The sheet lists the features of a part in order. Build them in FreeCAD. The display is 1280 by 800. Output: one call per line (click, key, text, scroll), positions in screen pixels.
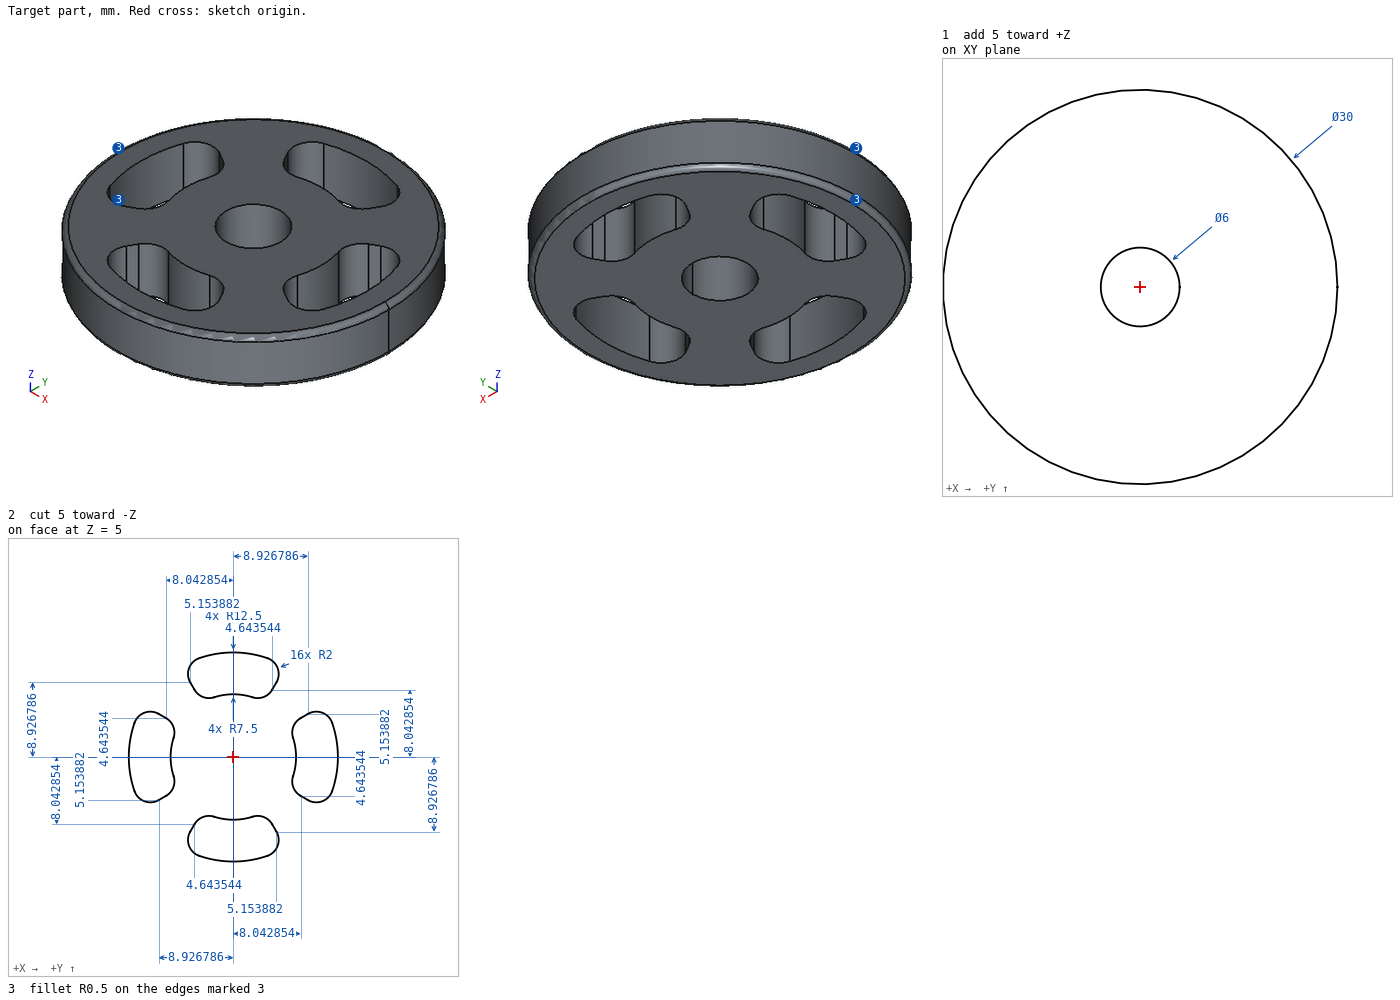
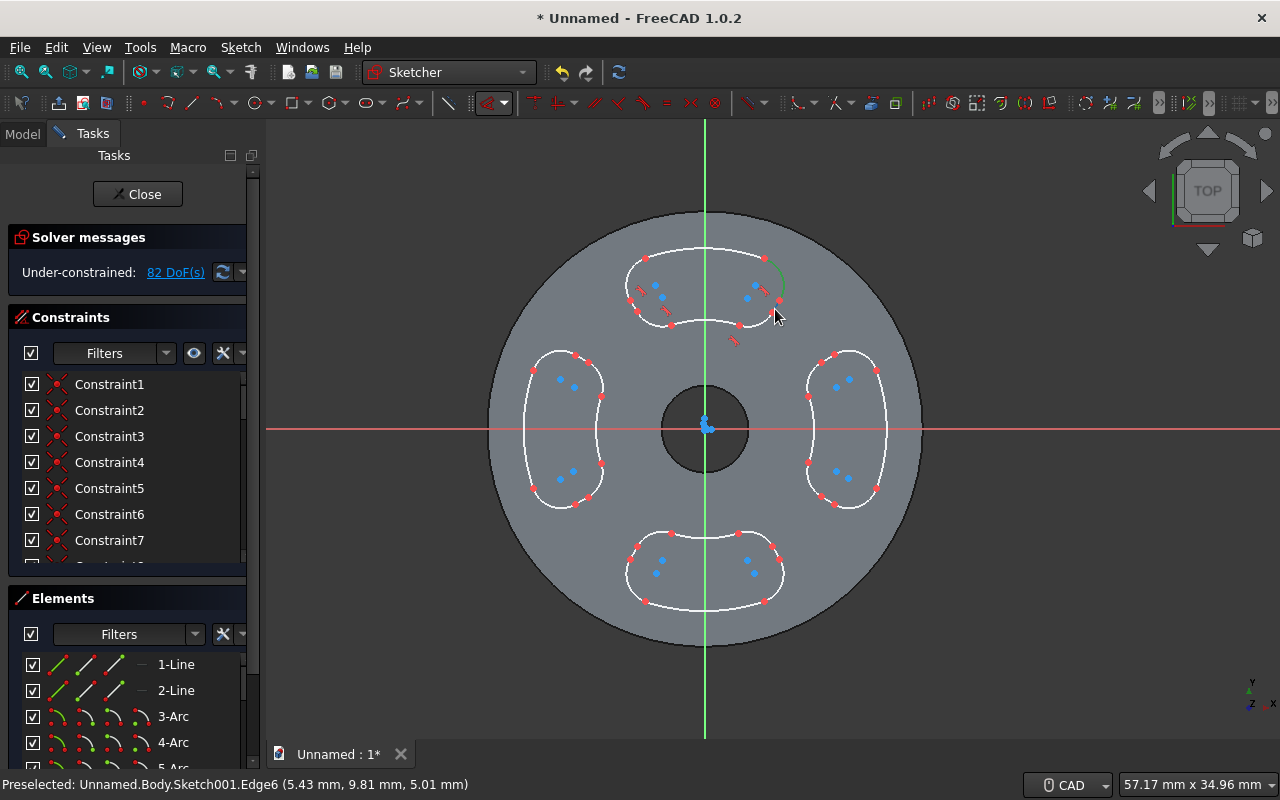
click(729, 250)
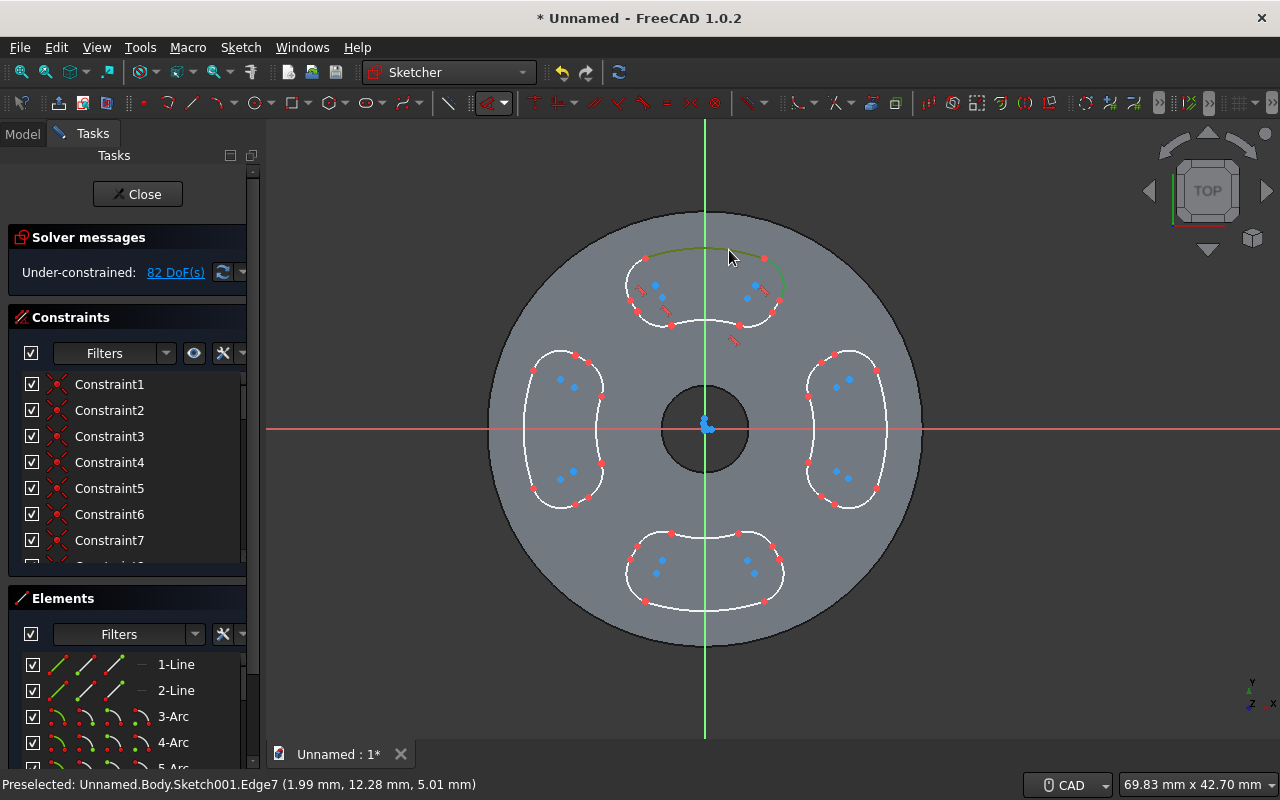
click(644, 104)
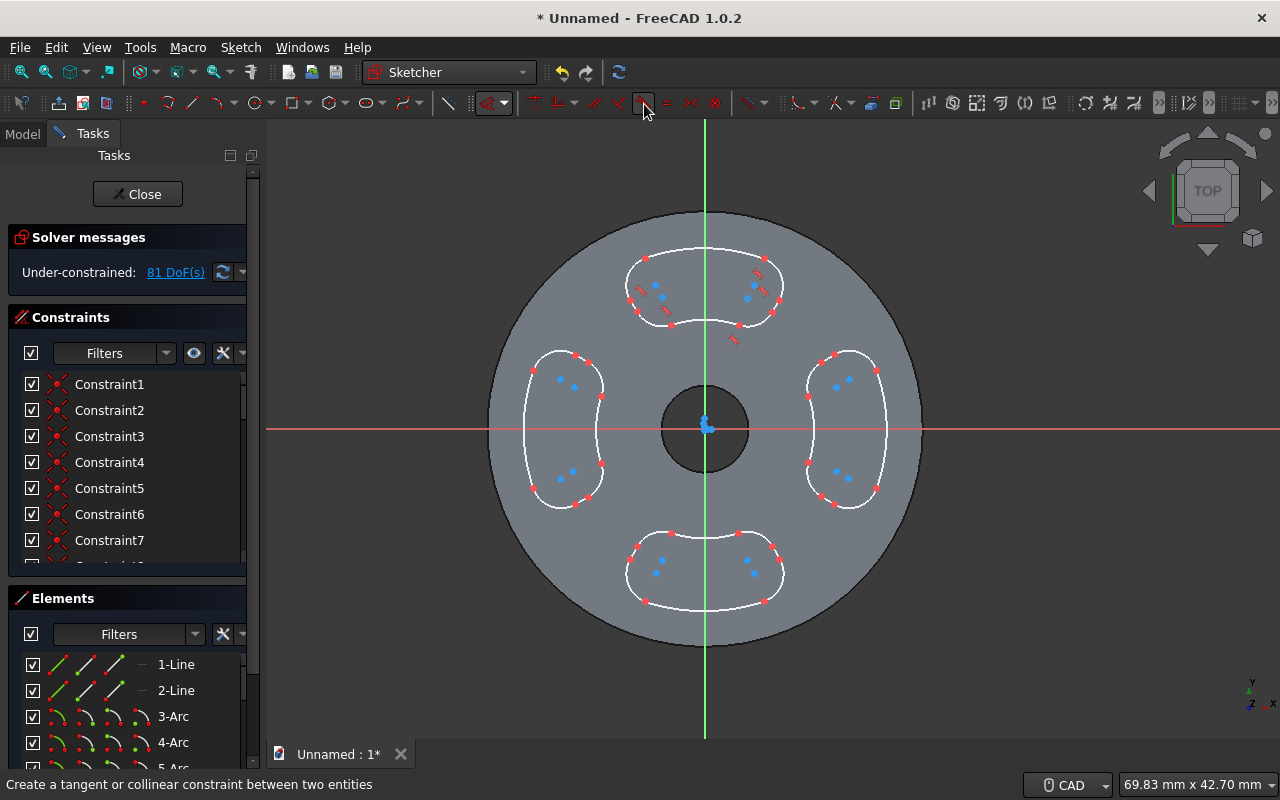
click(729, 250)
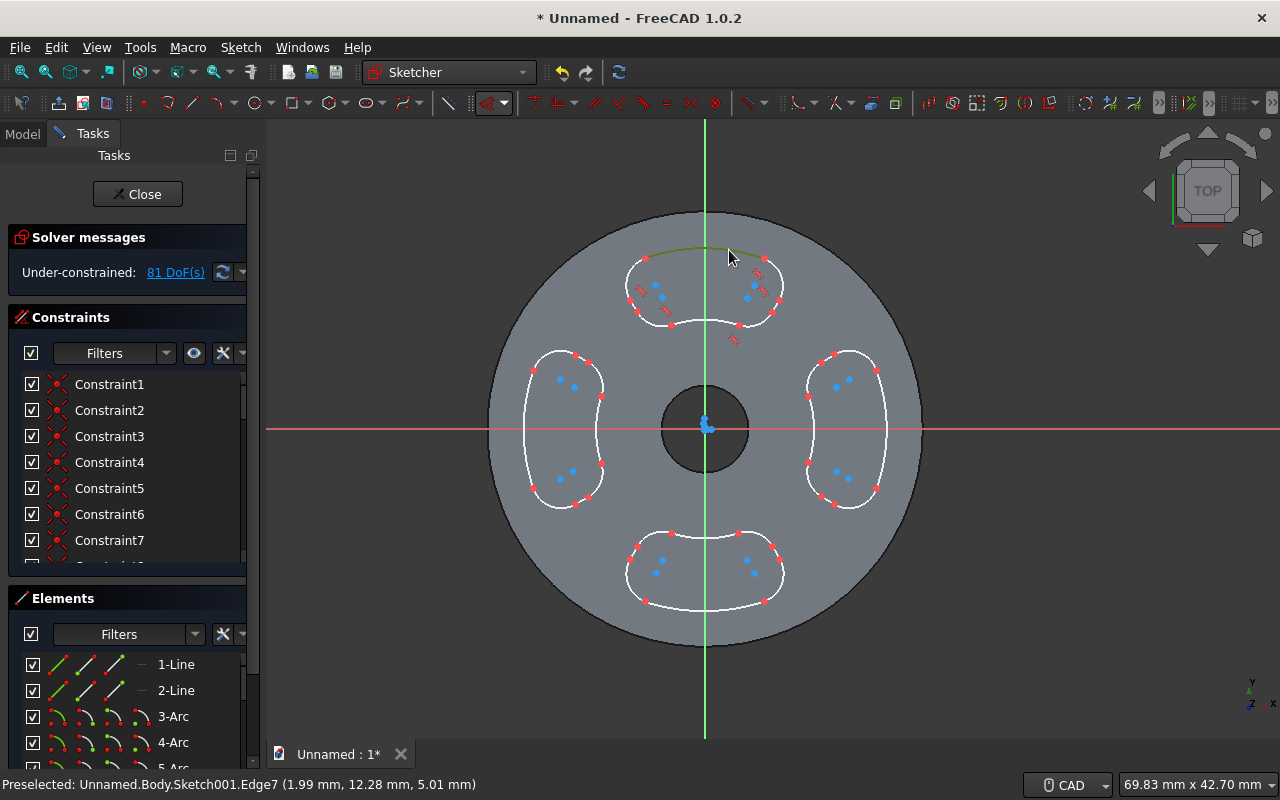
click(633, 267)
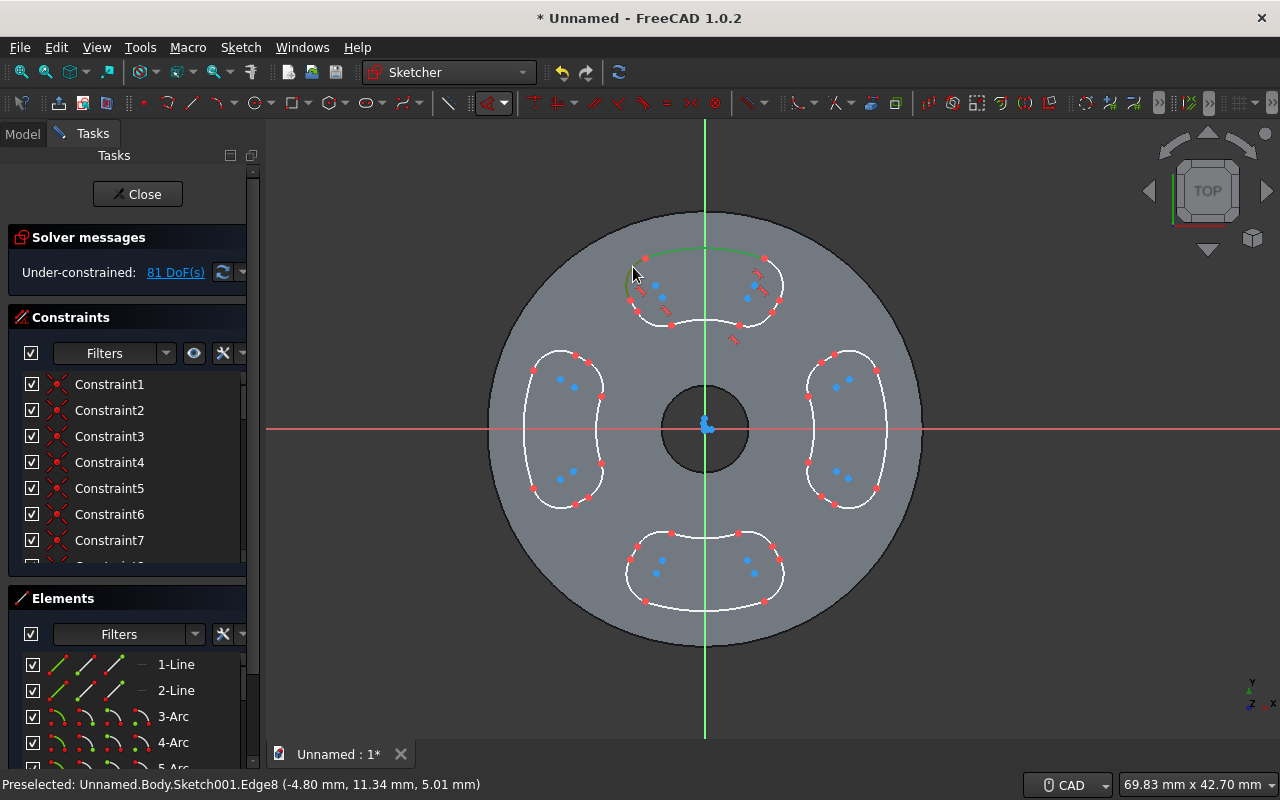
click(644, 104)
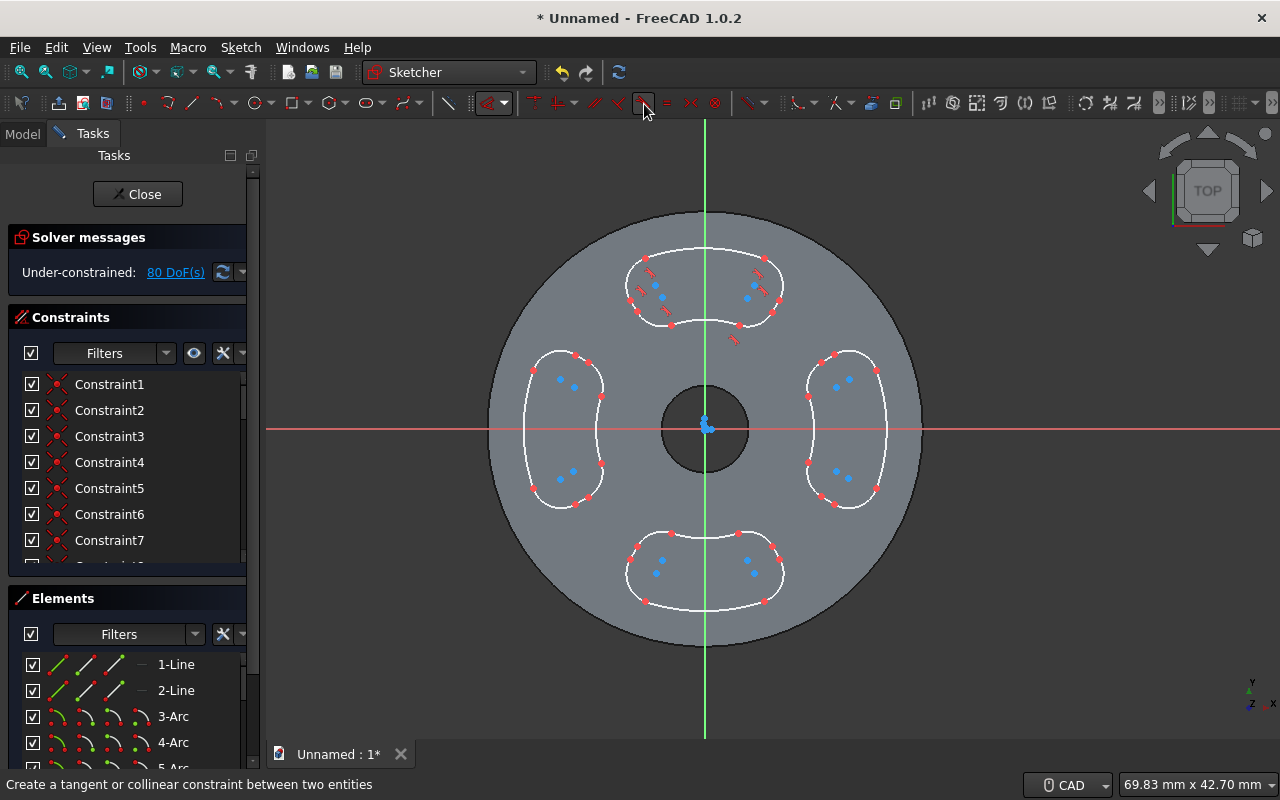
scroll(828, 359, up, 4)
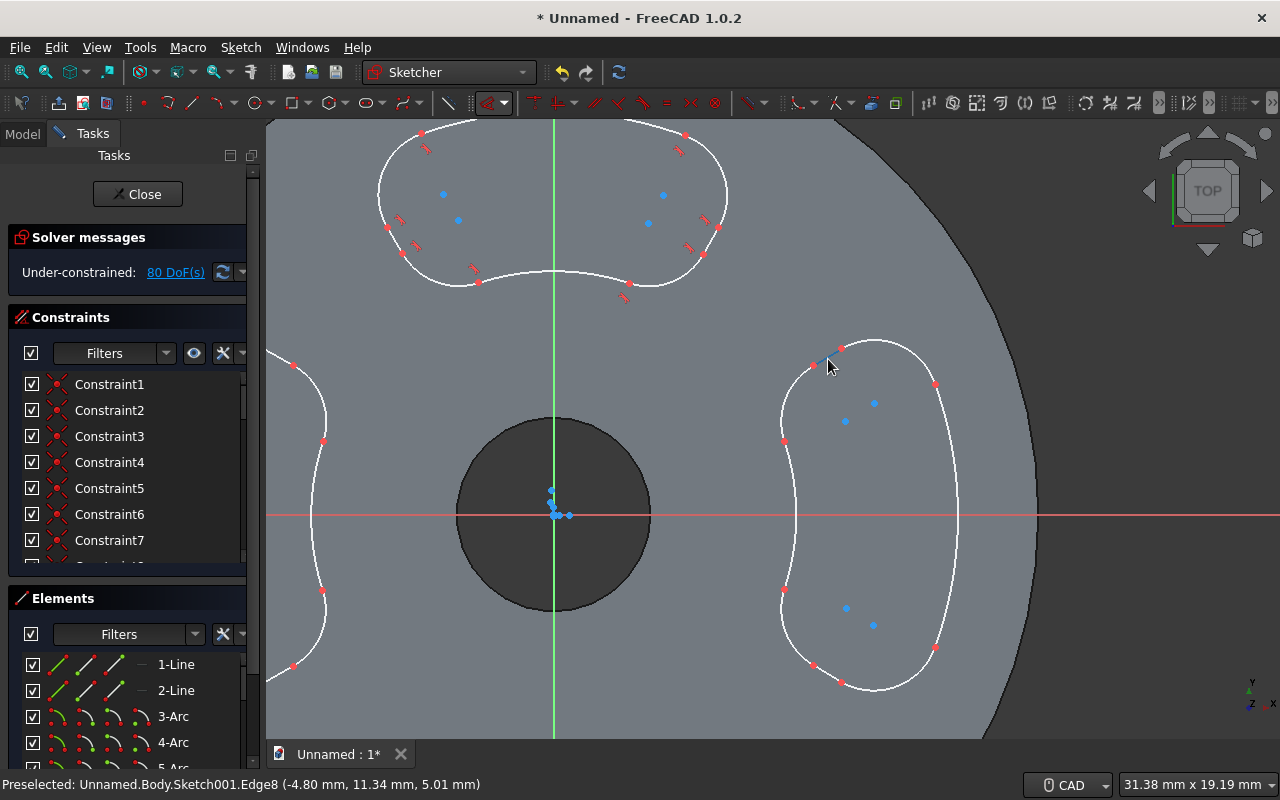
click(828, 357)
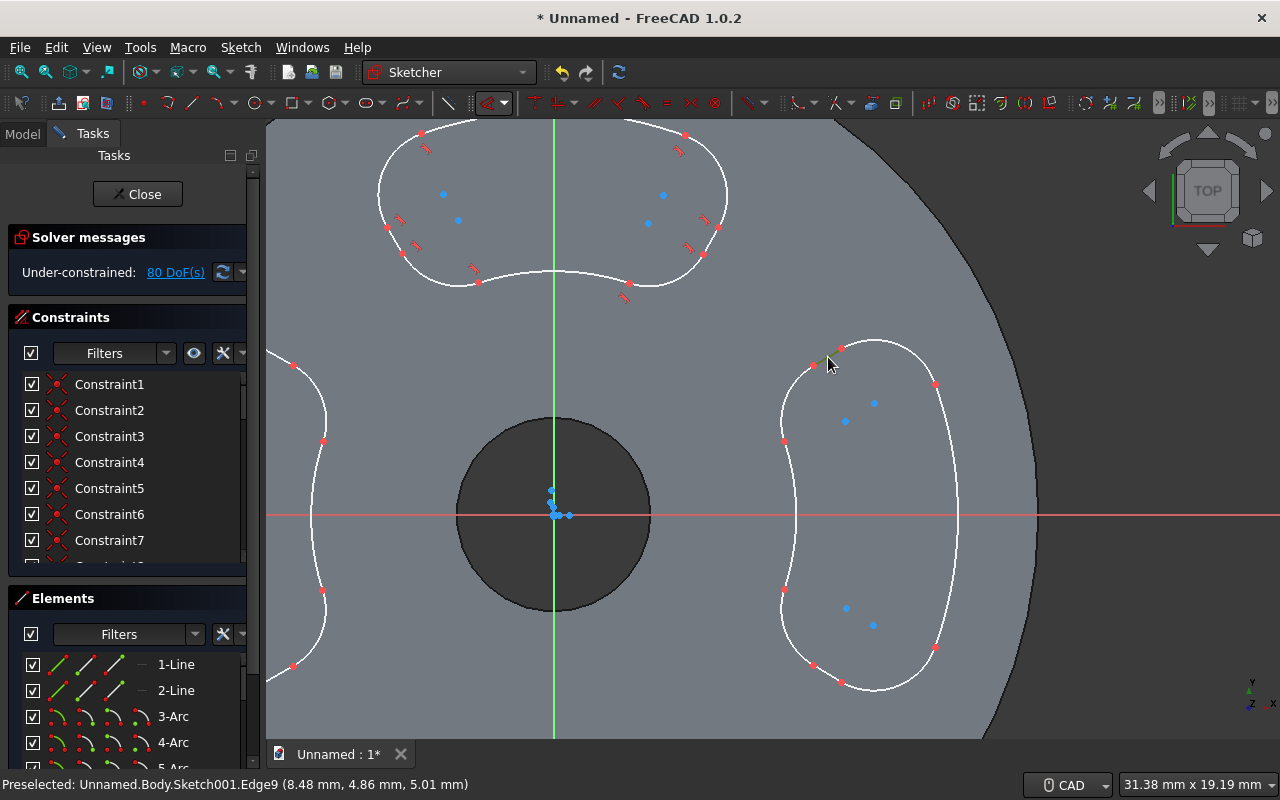
click(794, 383)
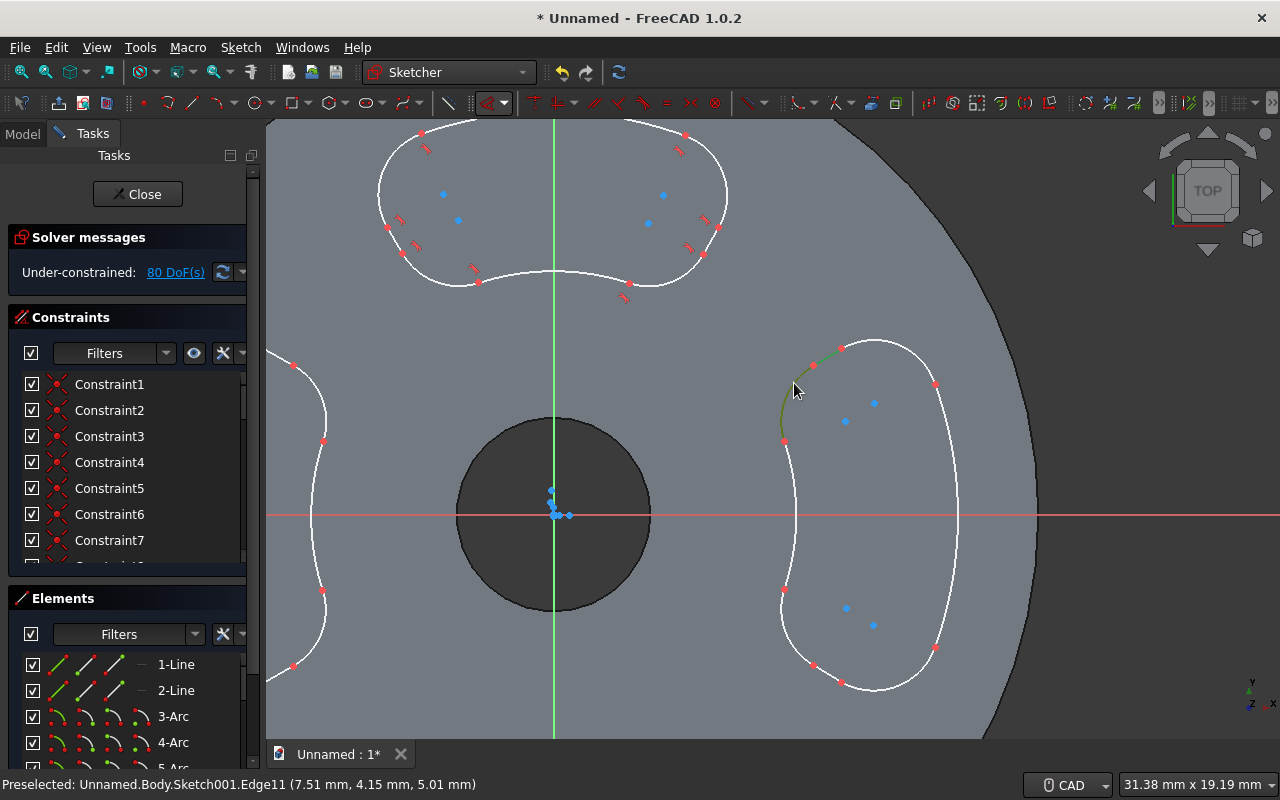
click(644, 104)